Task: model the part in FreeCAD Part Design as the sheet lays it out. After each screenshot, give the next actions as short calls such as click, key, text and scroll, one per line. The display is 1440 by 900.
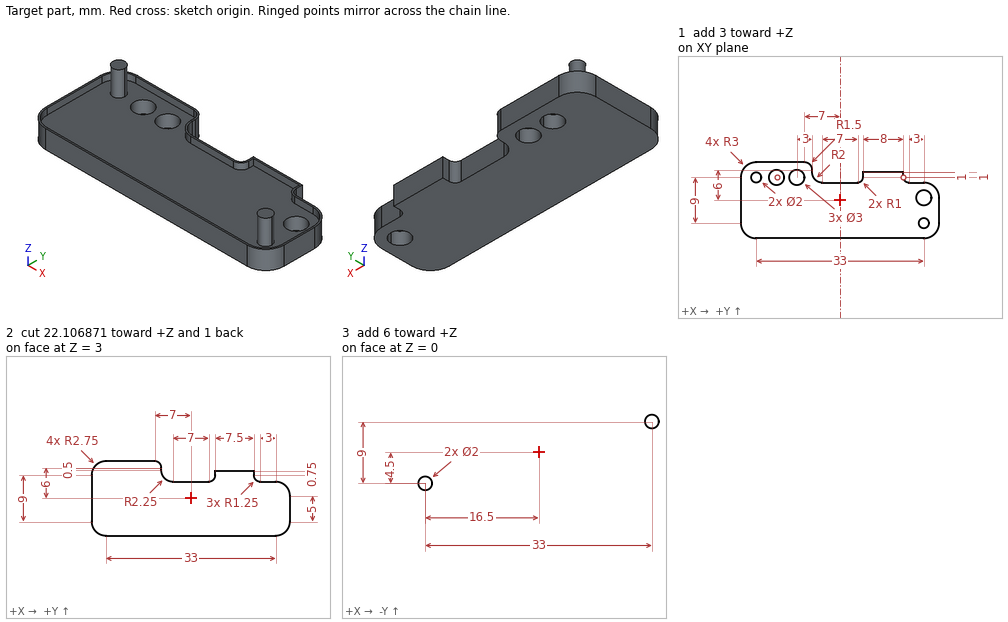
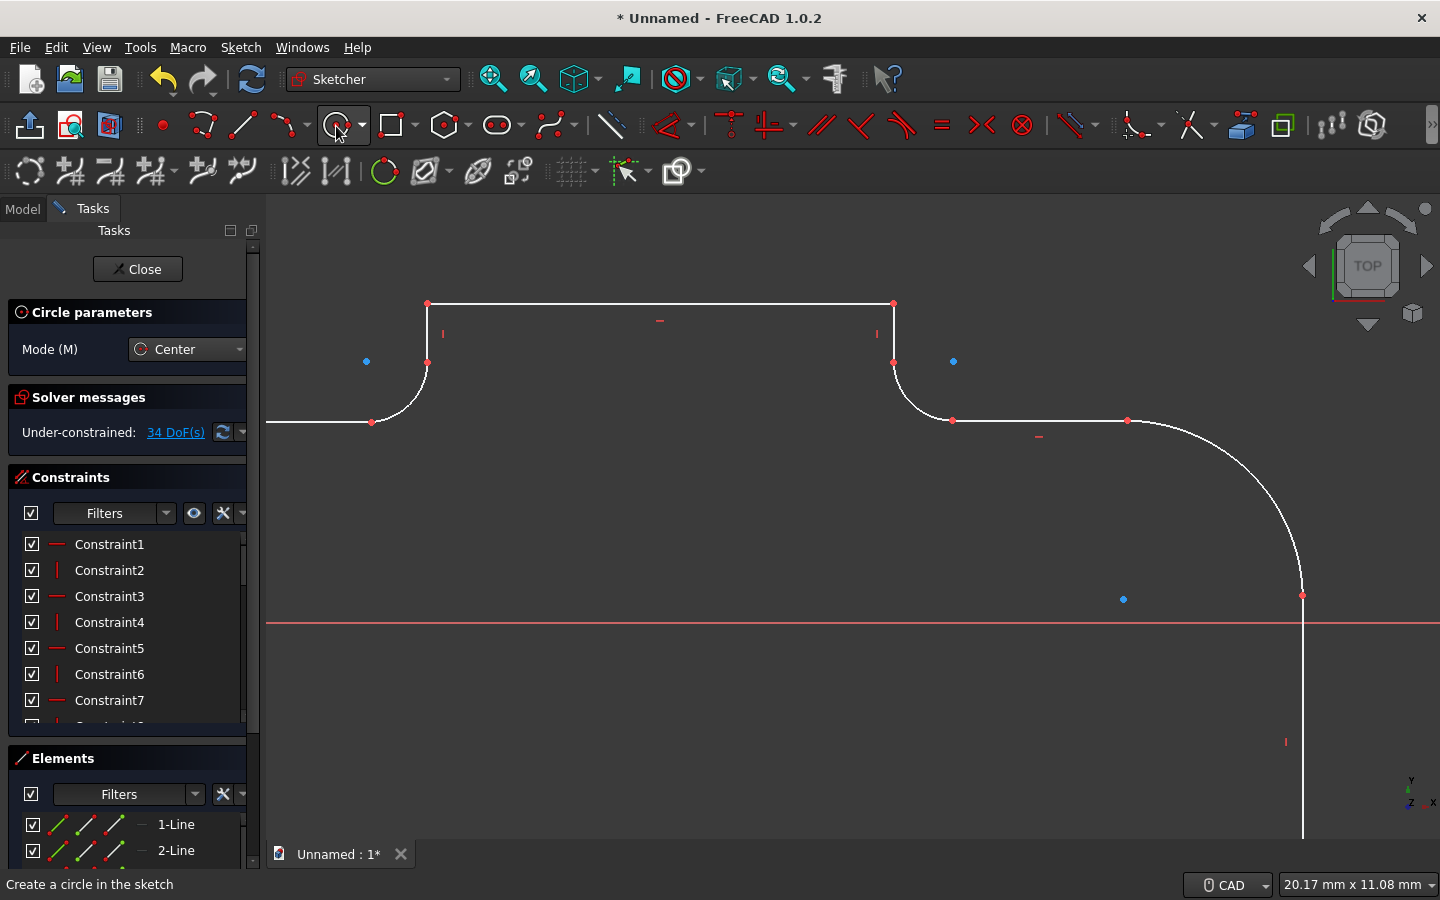
scroll(1051, 471, down, 6)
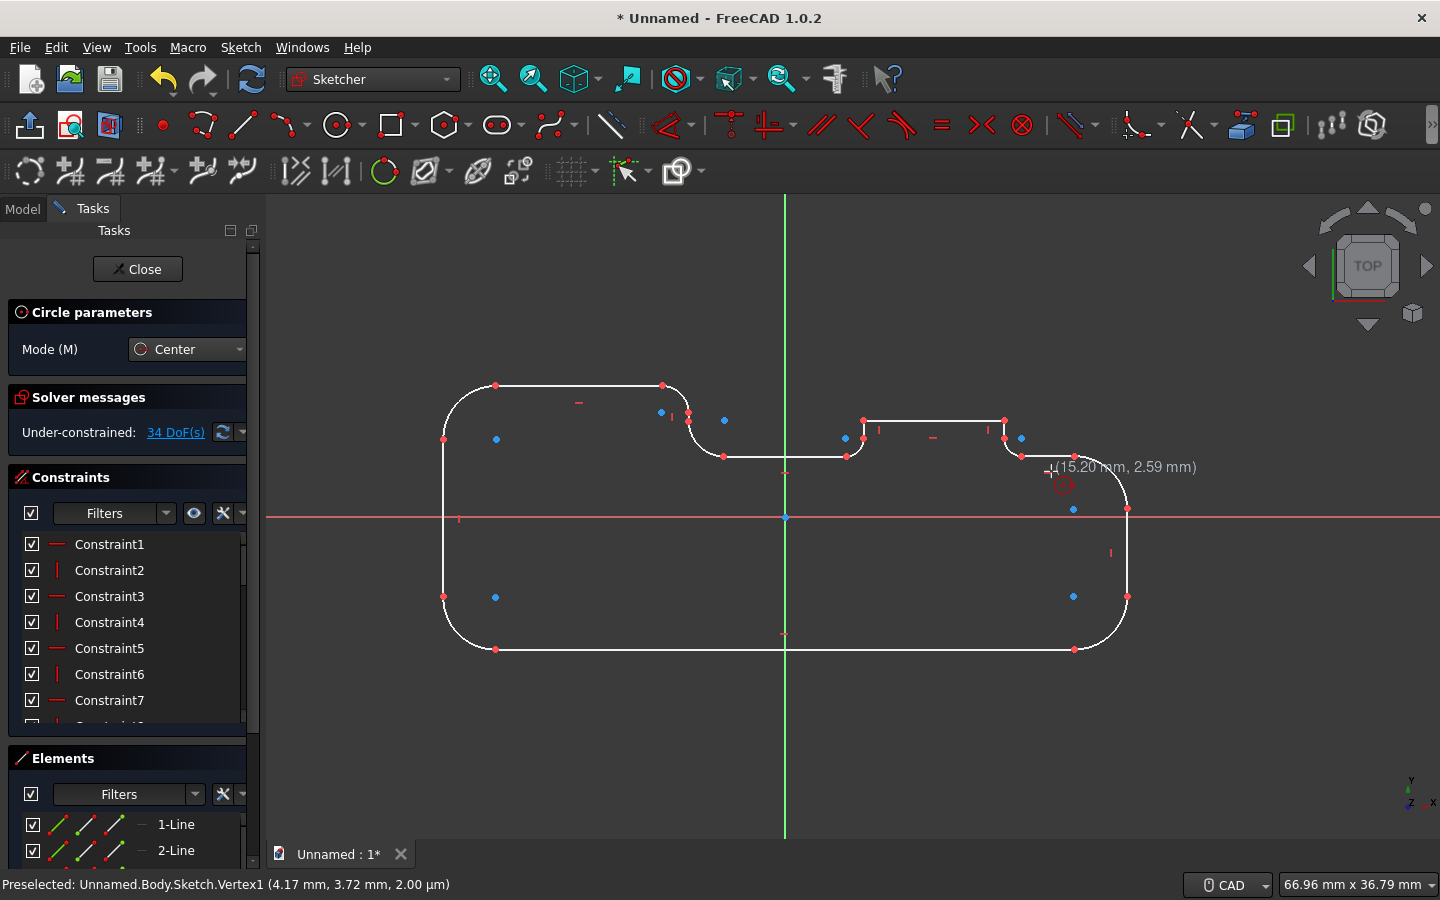
scroll(1074, 596, up, 2)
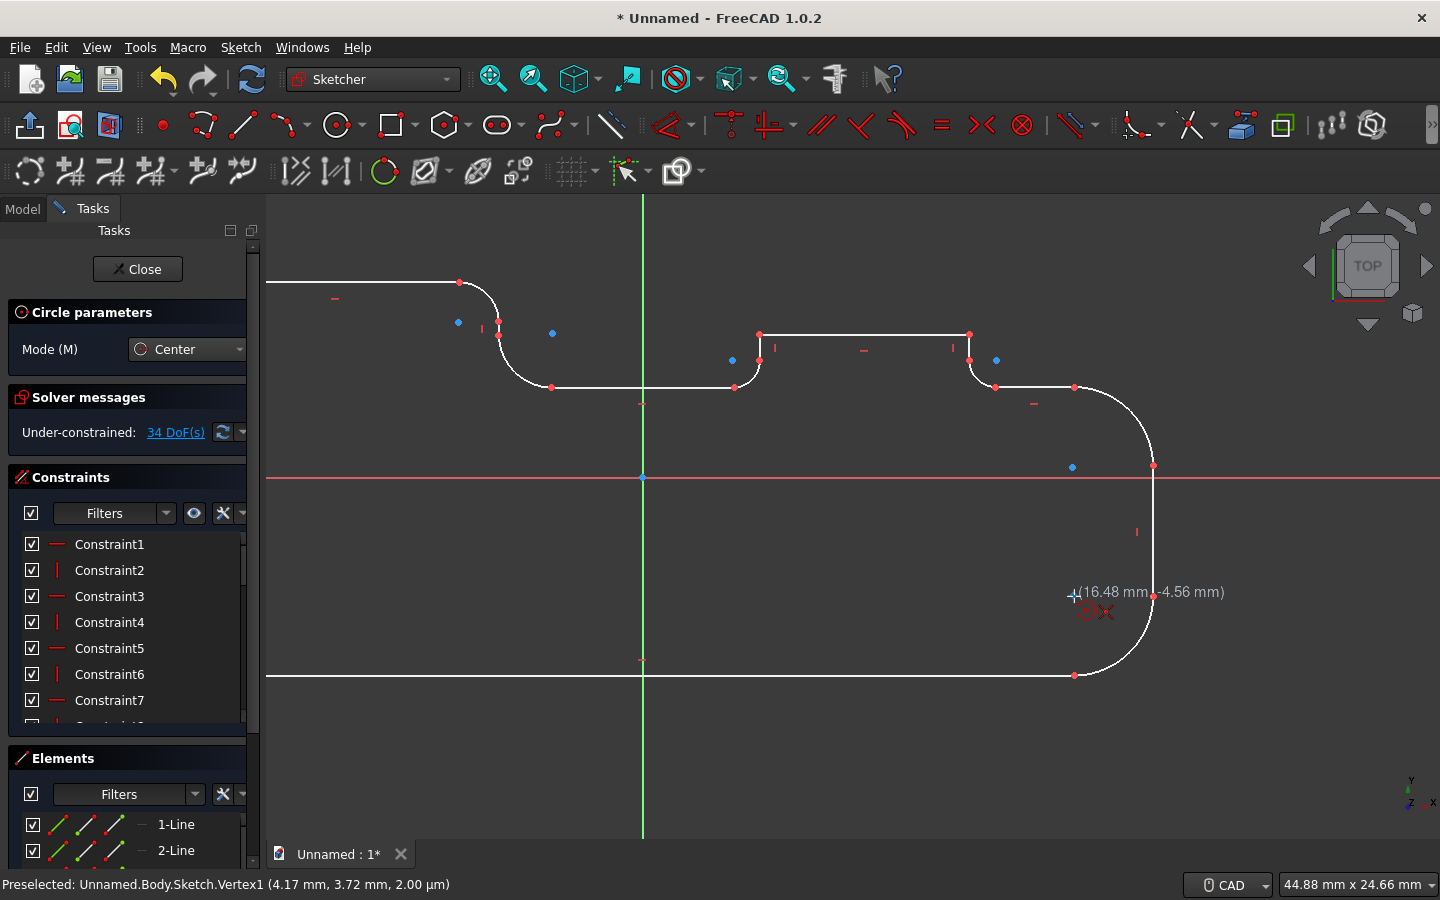
click(1074, 596)
move(1093, 577)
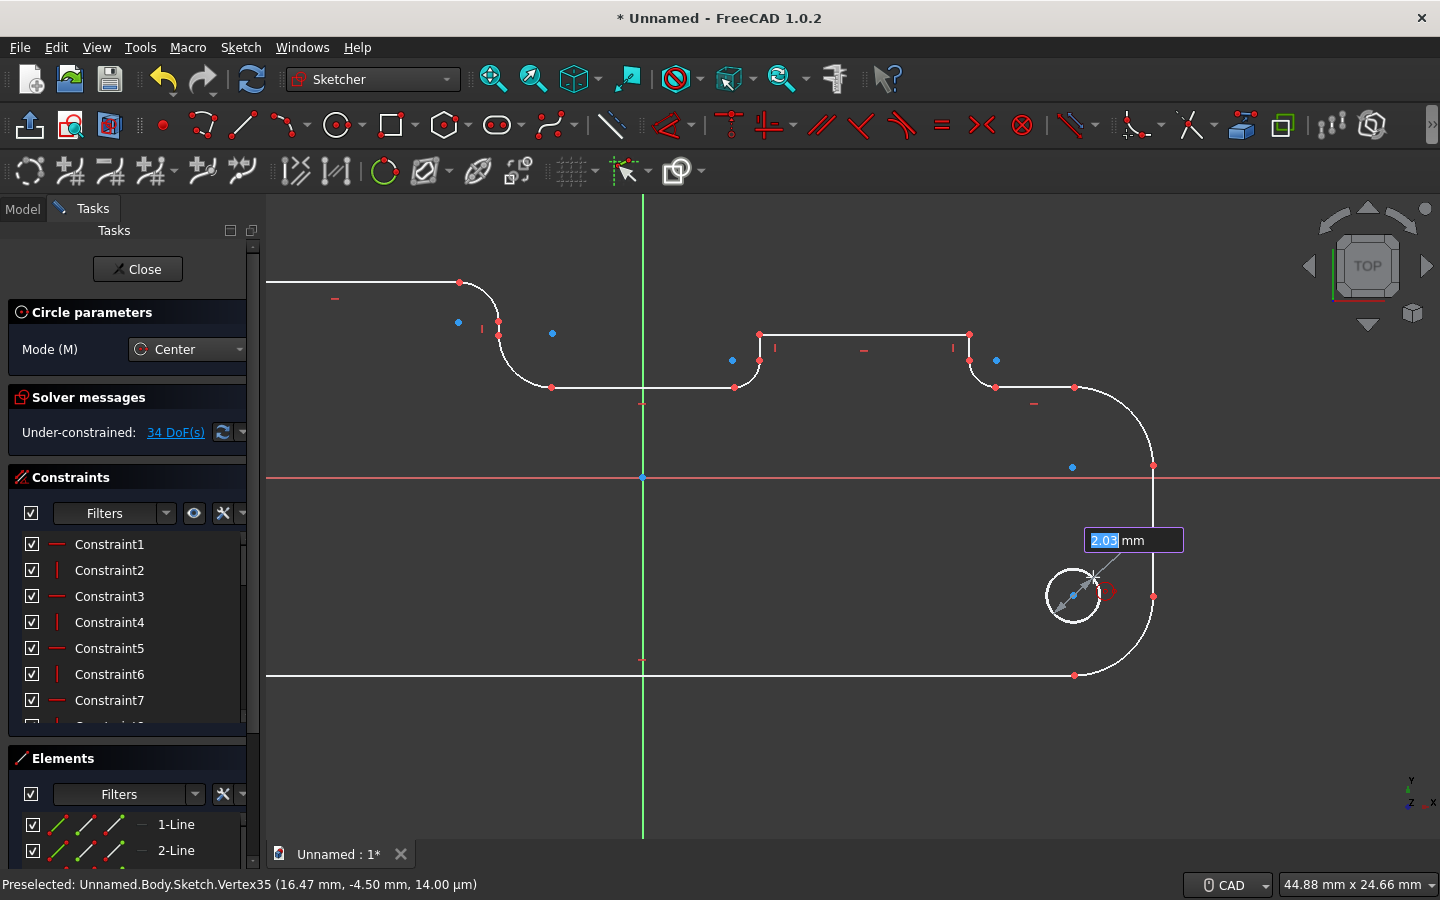
text(2)
key(Return)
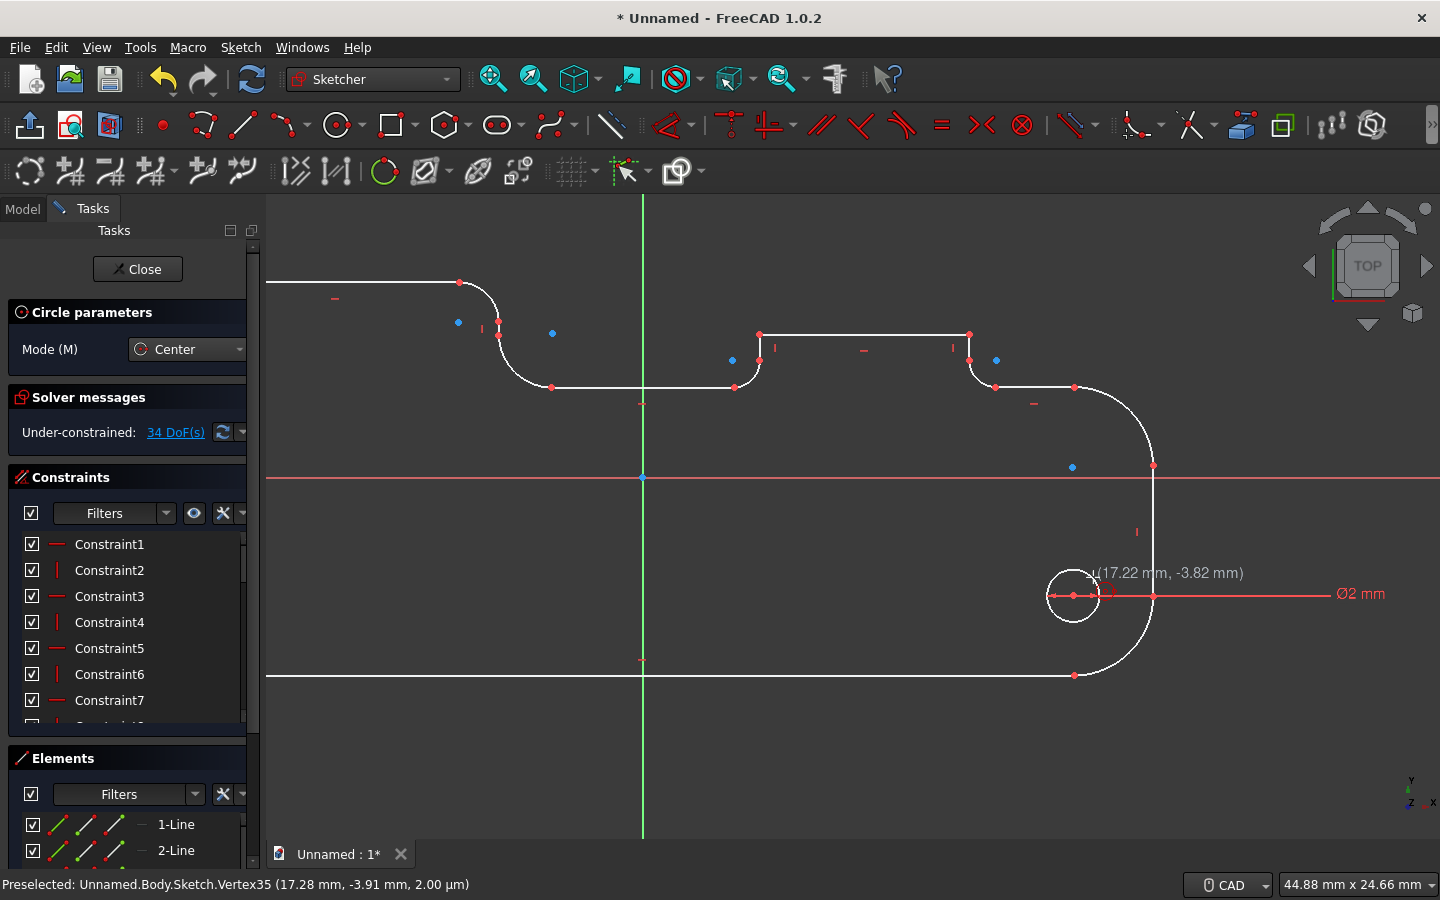
click(1074, 465)
move(1102, 437)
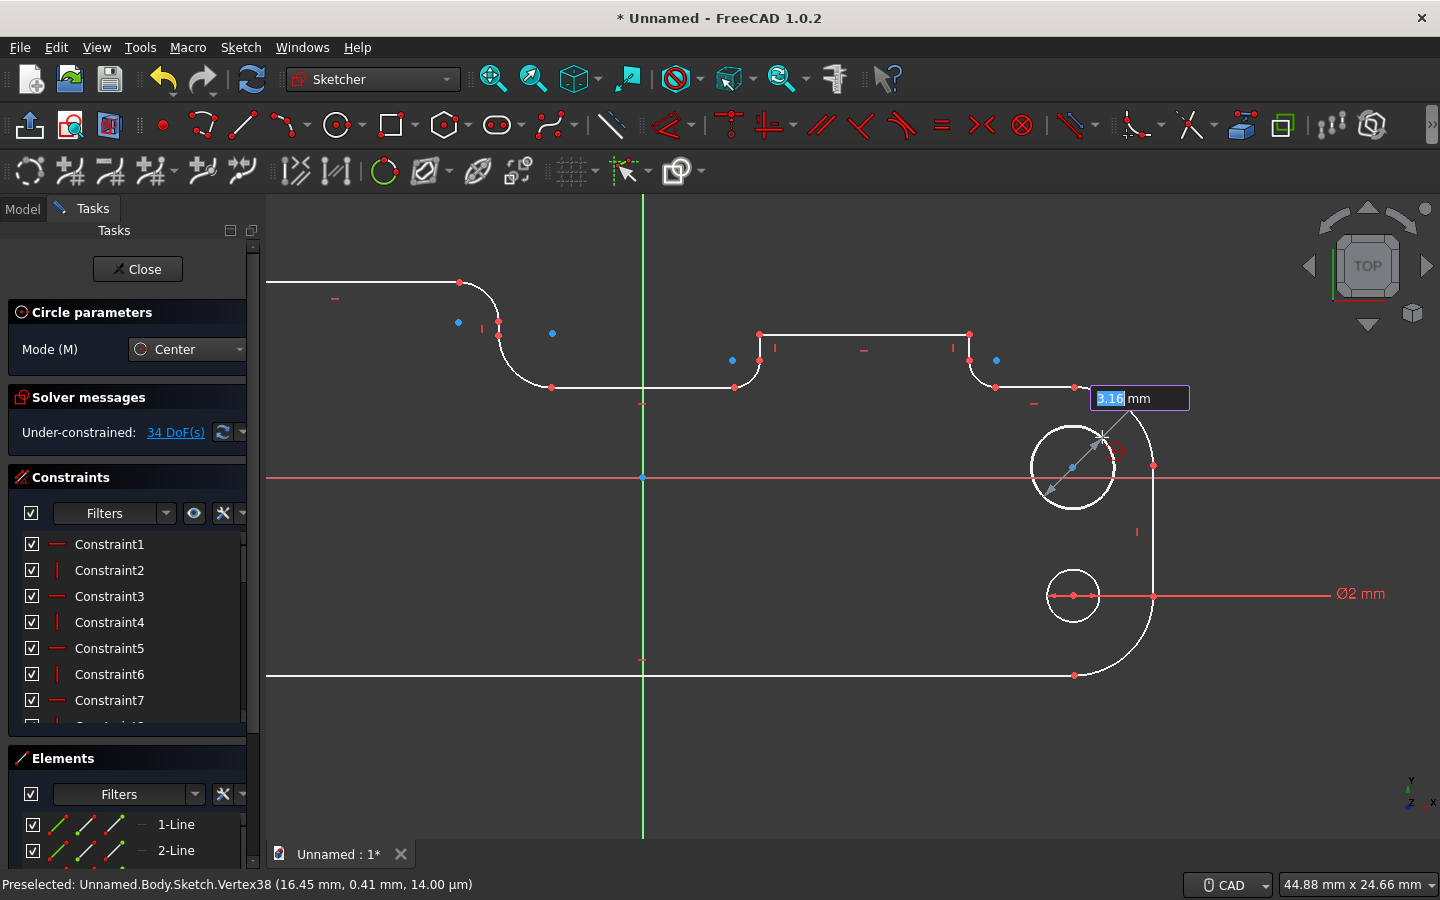
text(3)
key(Return)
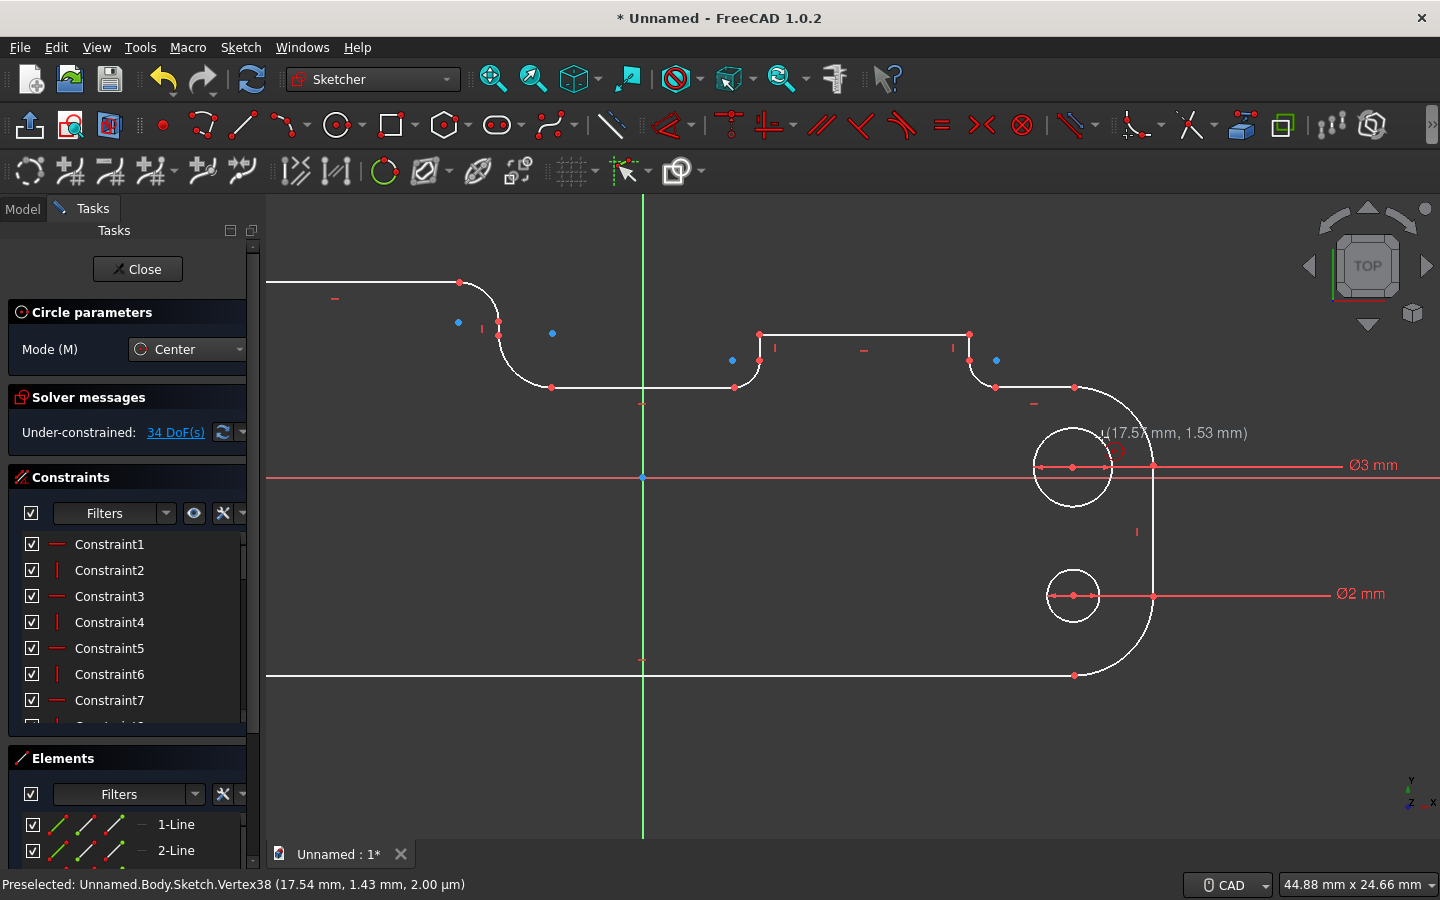
click(420, 360)
move(448, 333)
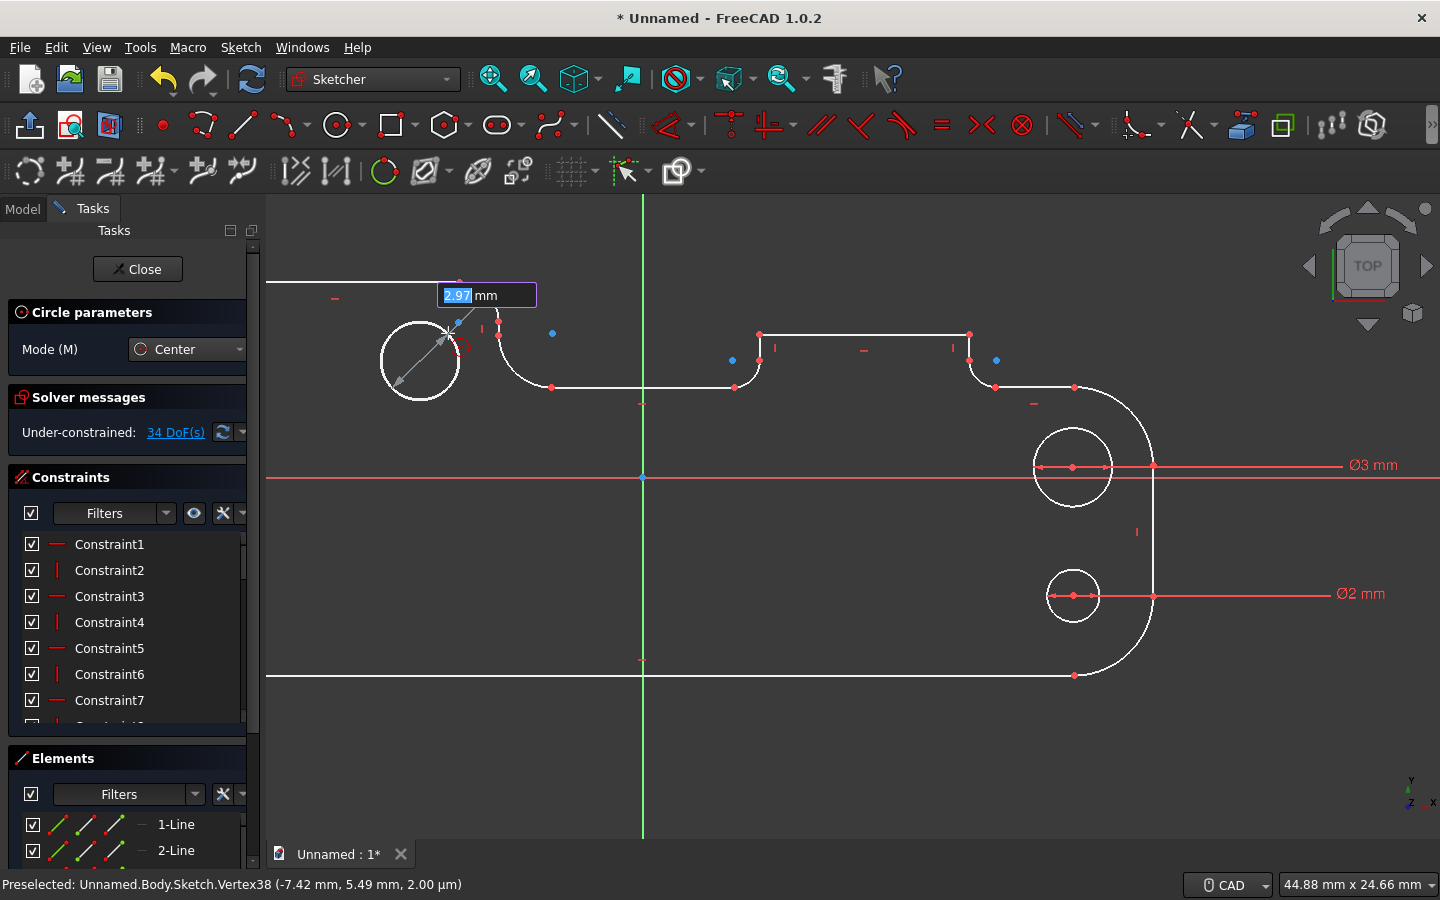
text(3)
key(Return)